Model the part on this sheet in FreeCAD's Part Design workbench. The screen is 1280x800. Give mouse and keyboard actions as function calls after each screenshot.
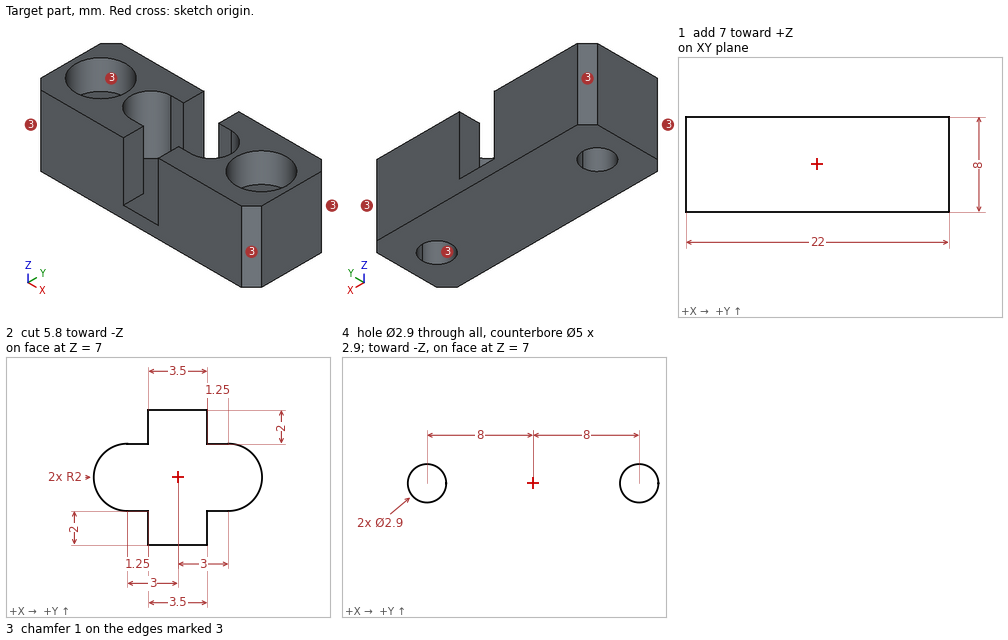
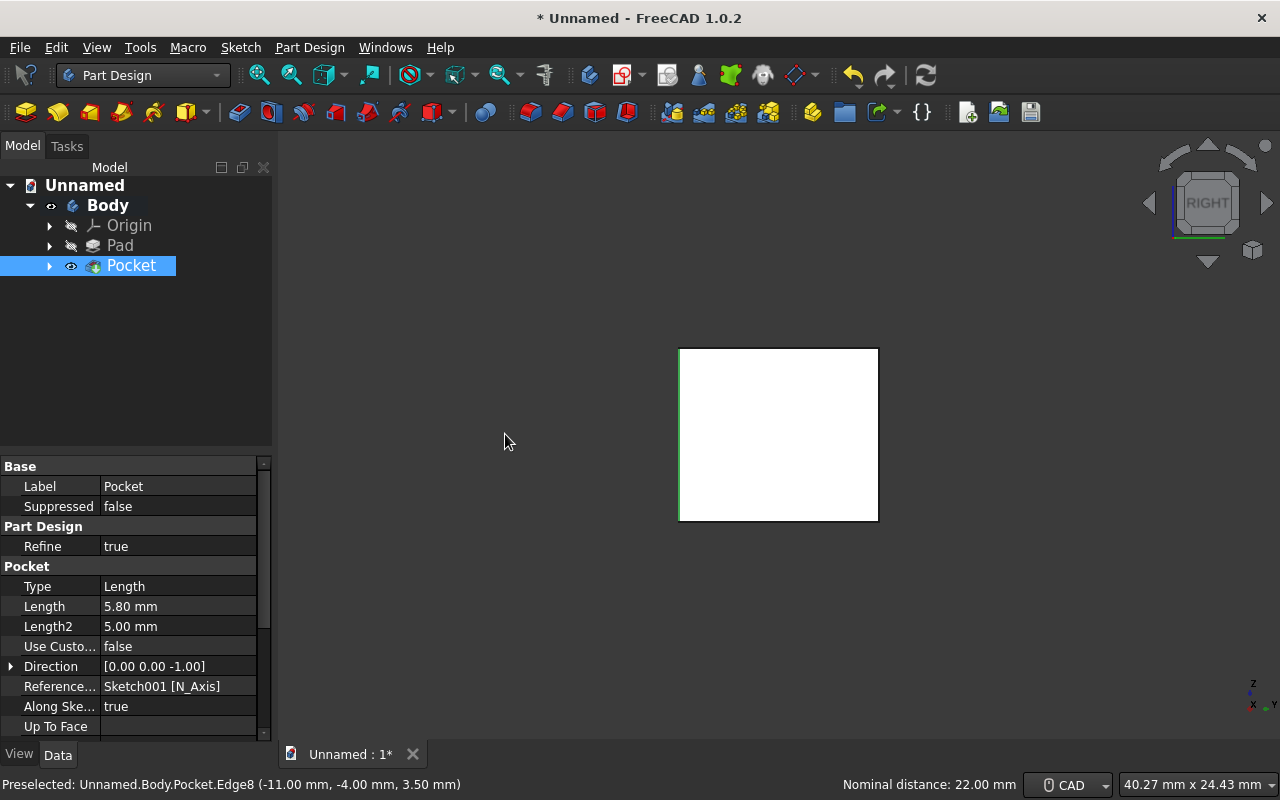
click(260, 76)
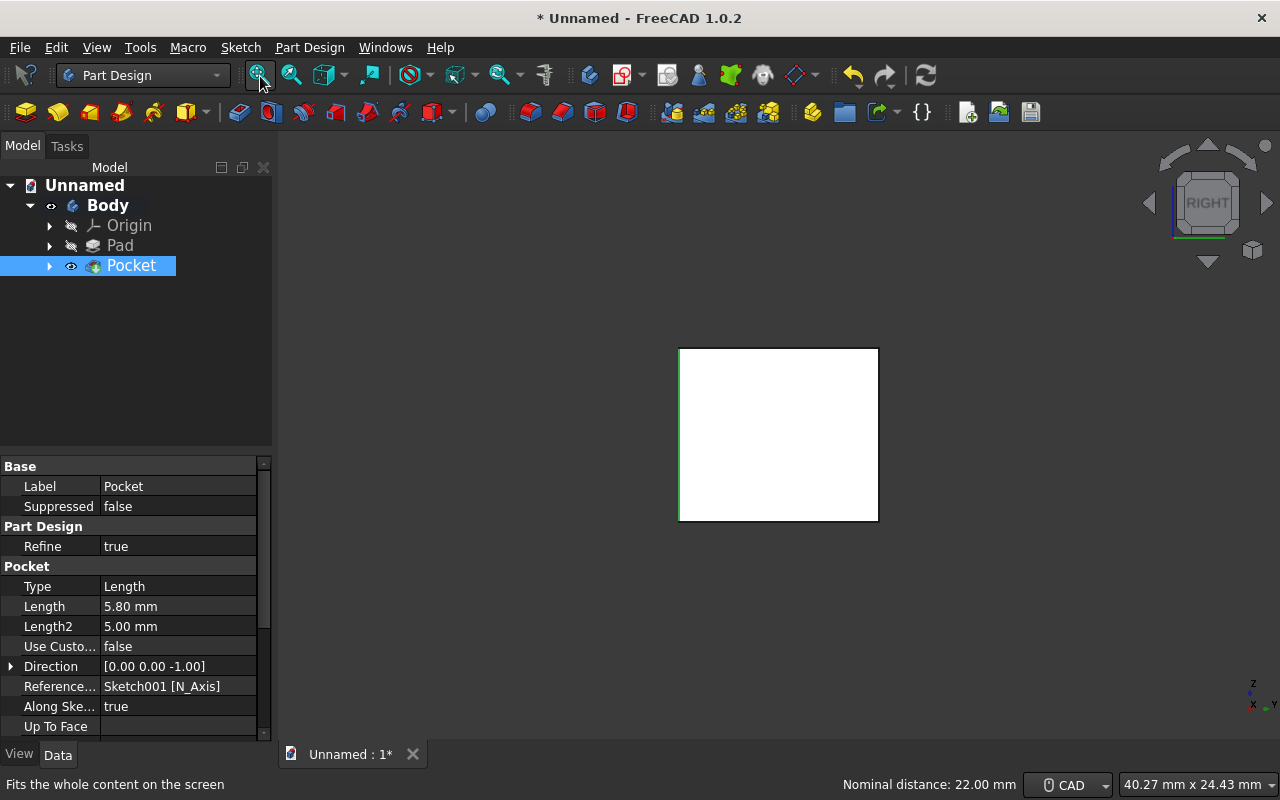
click(879, 434, ctrl)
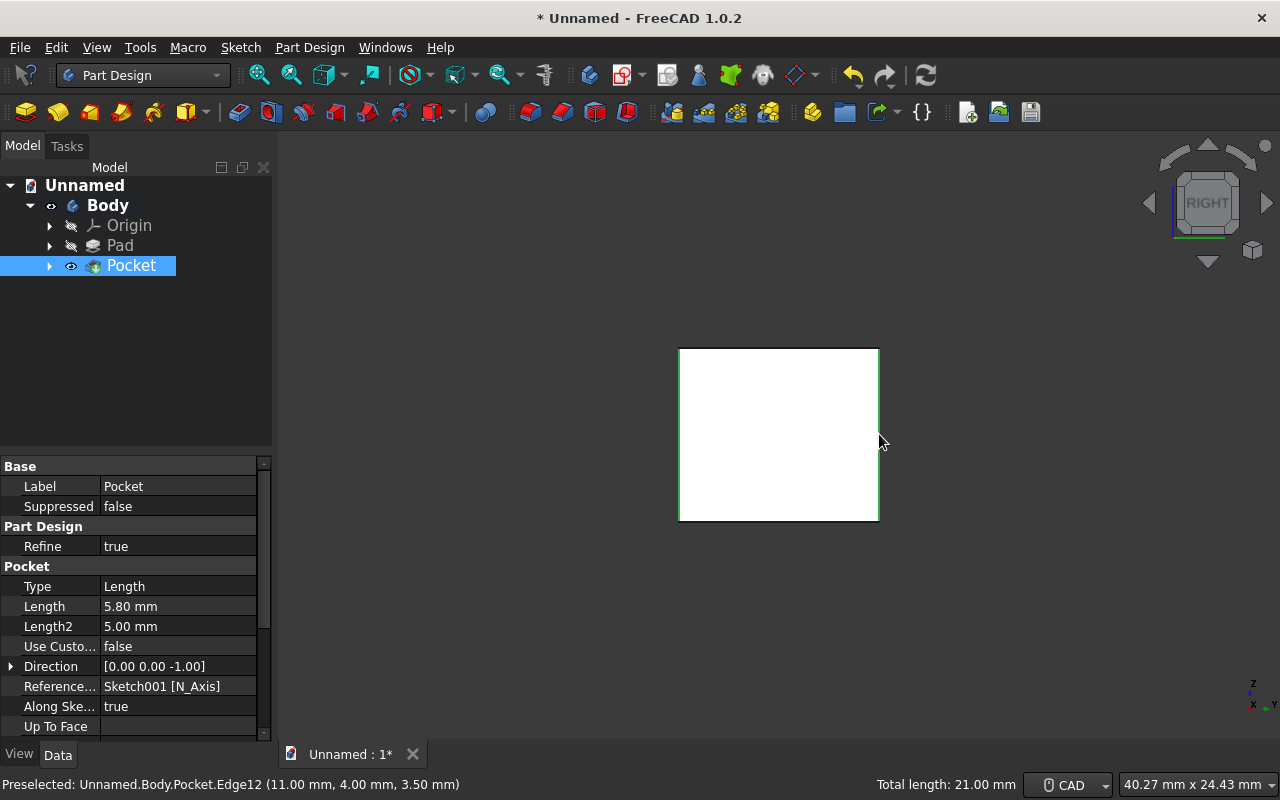
key(5)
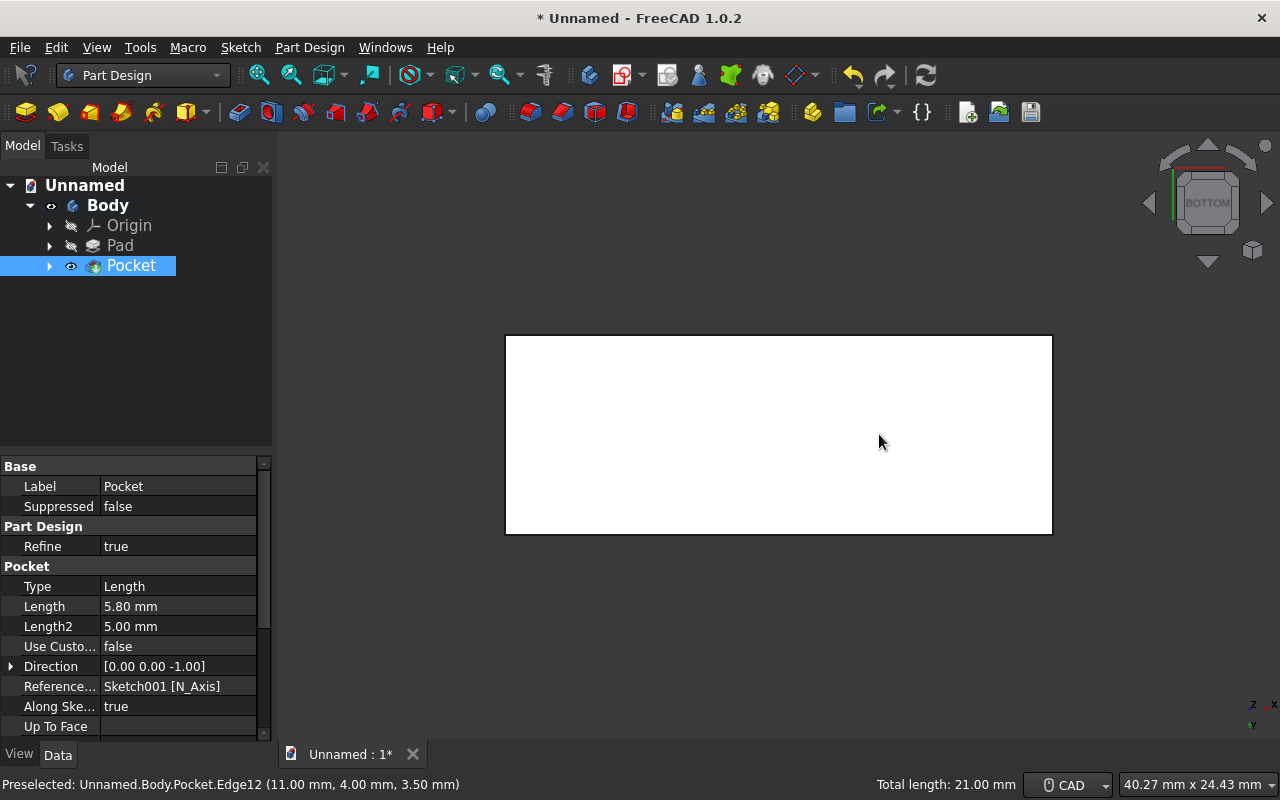
key(4)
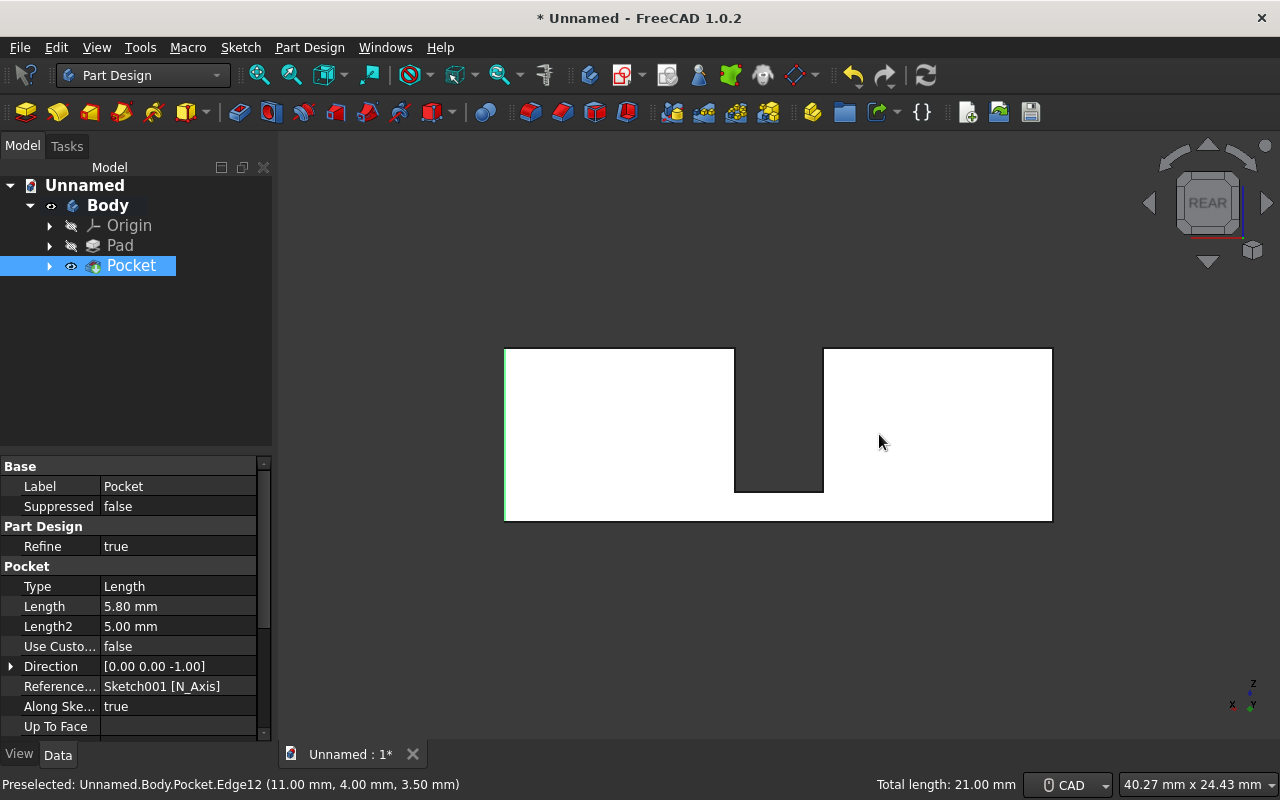
click(1053, 434, ctrl)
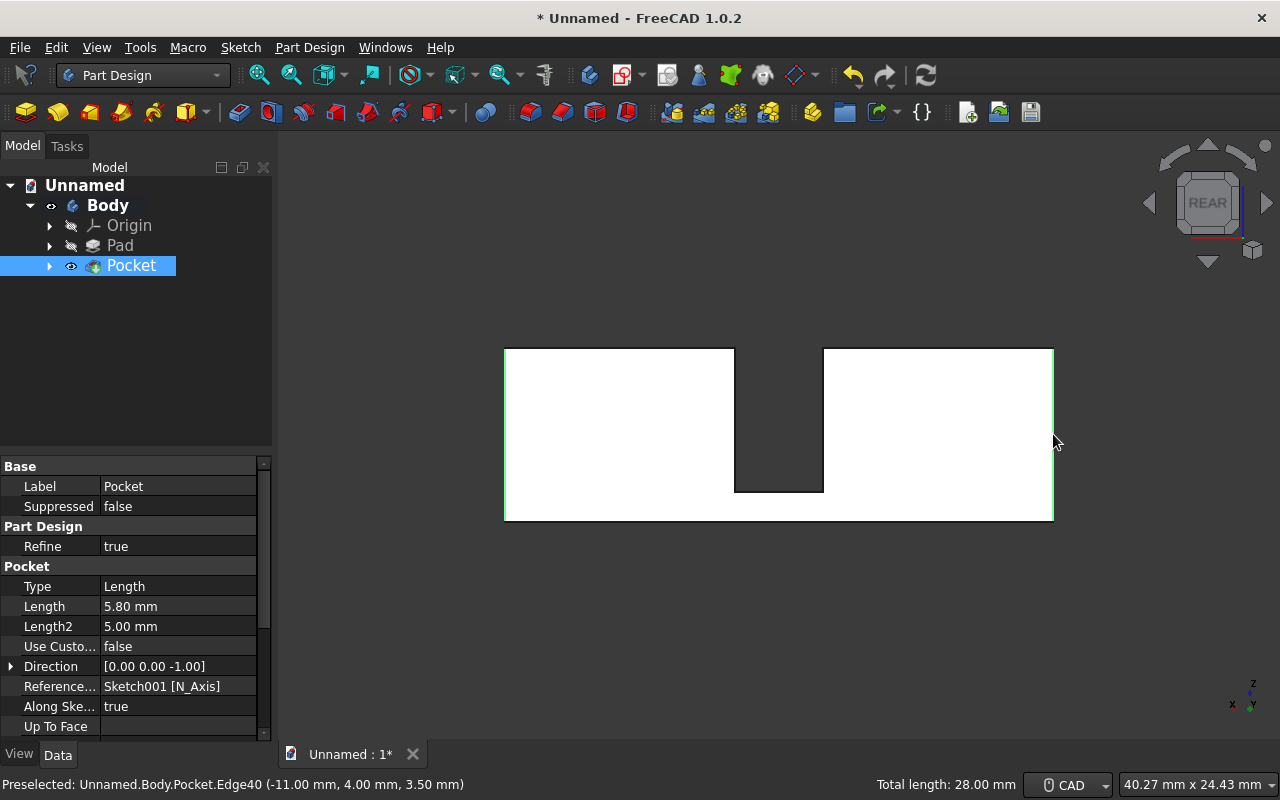
click(564, 112)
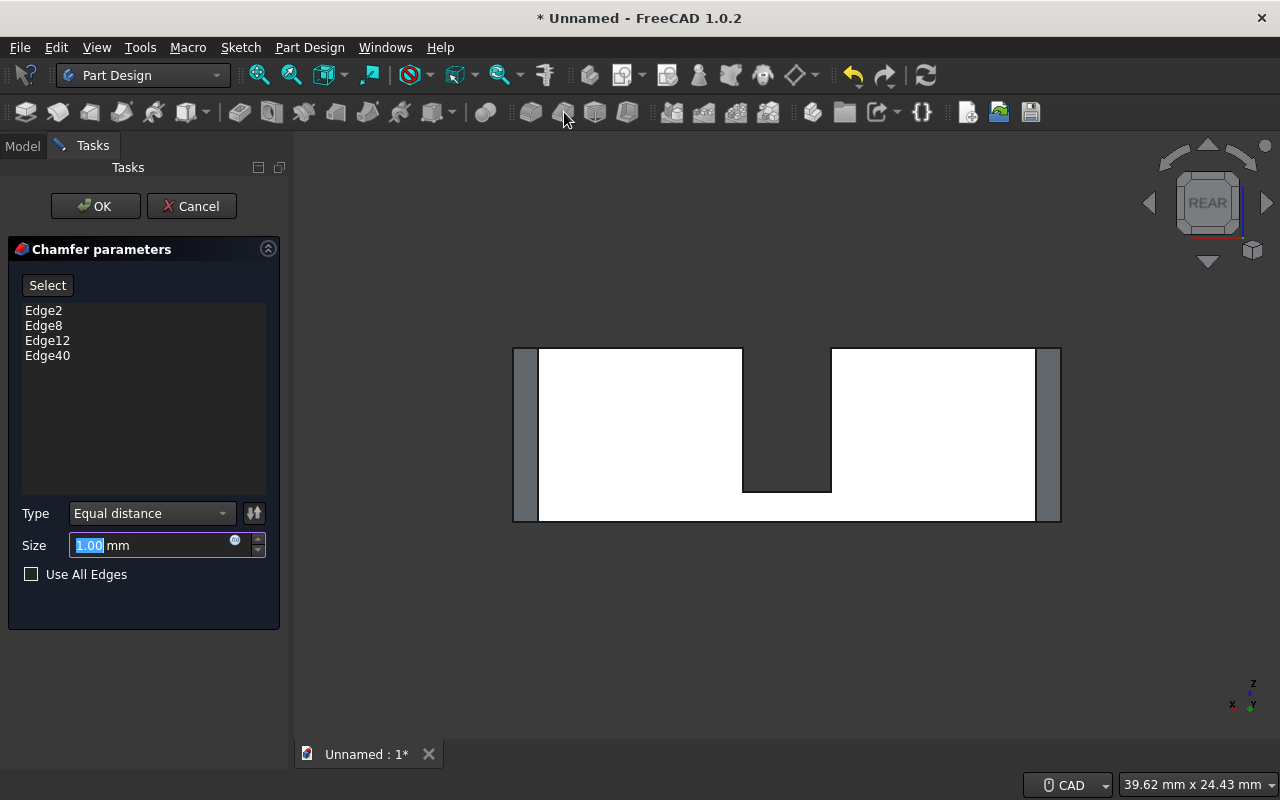
text(1)
key(Tab)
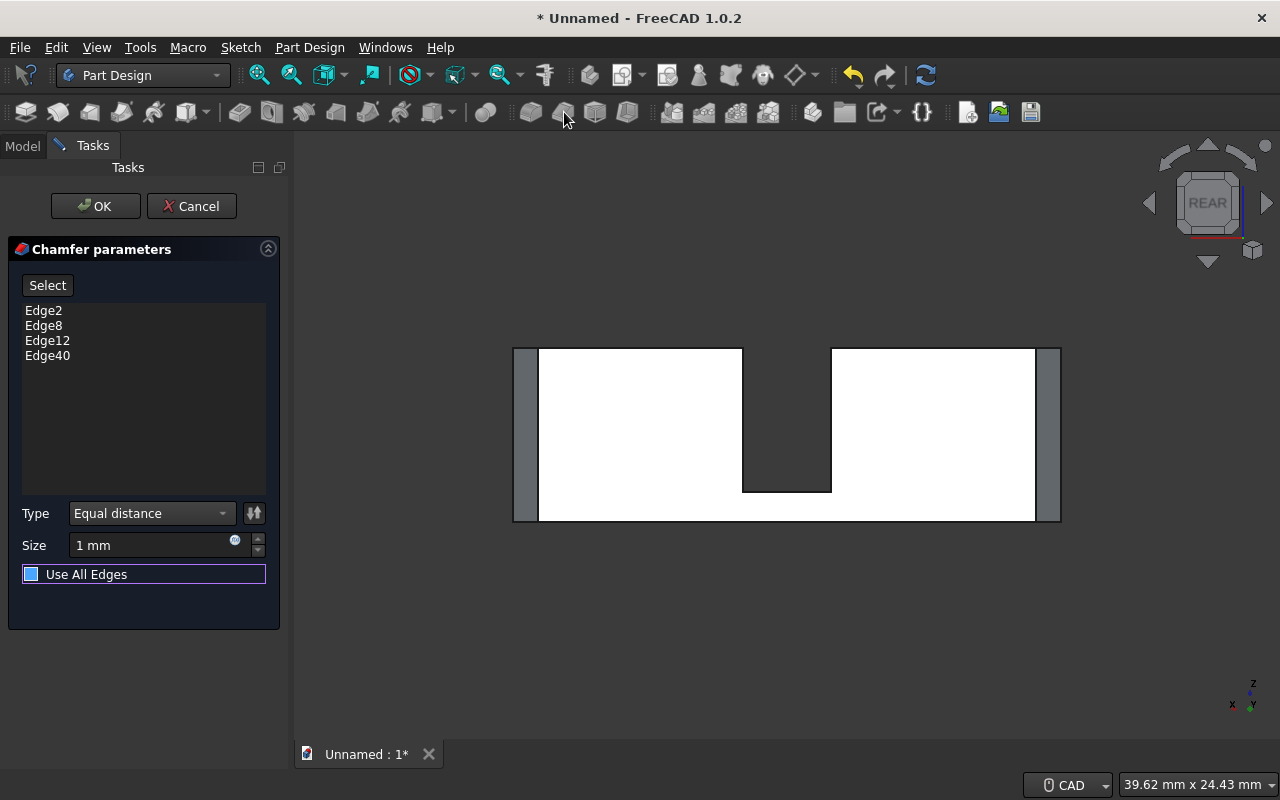
click(96, 206)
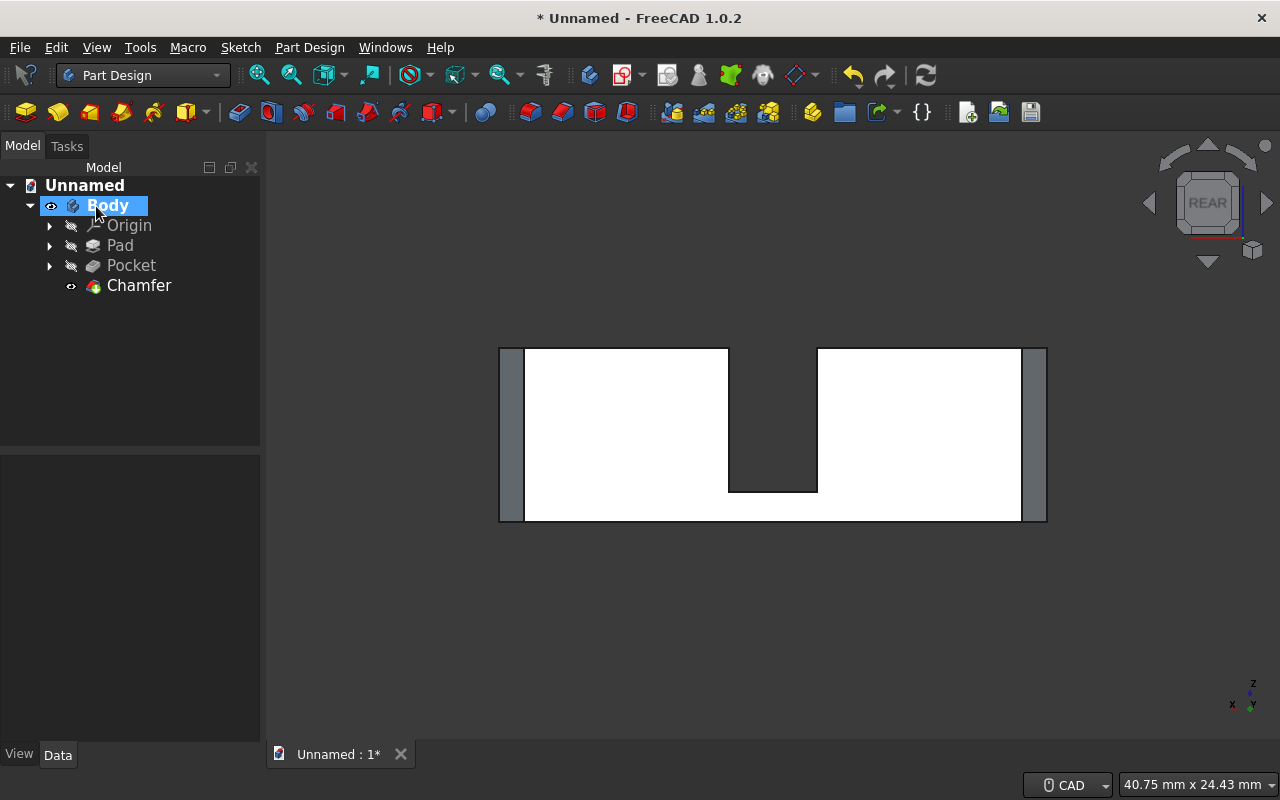
key(0)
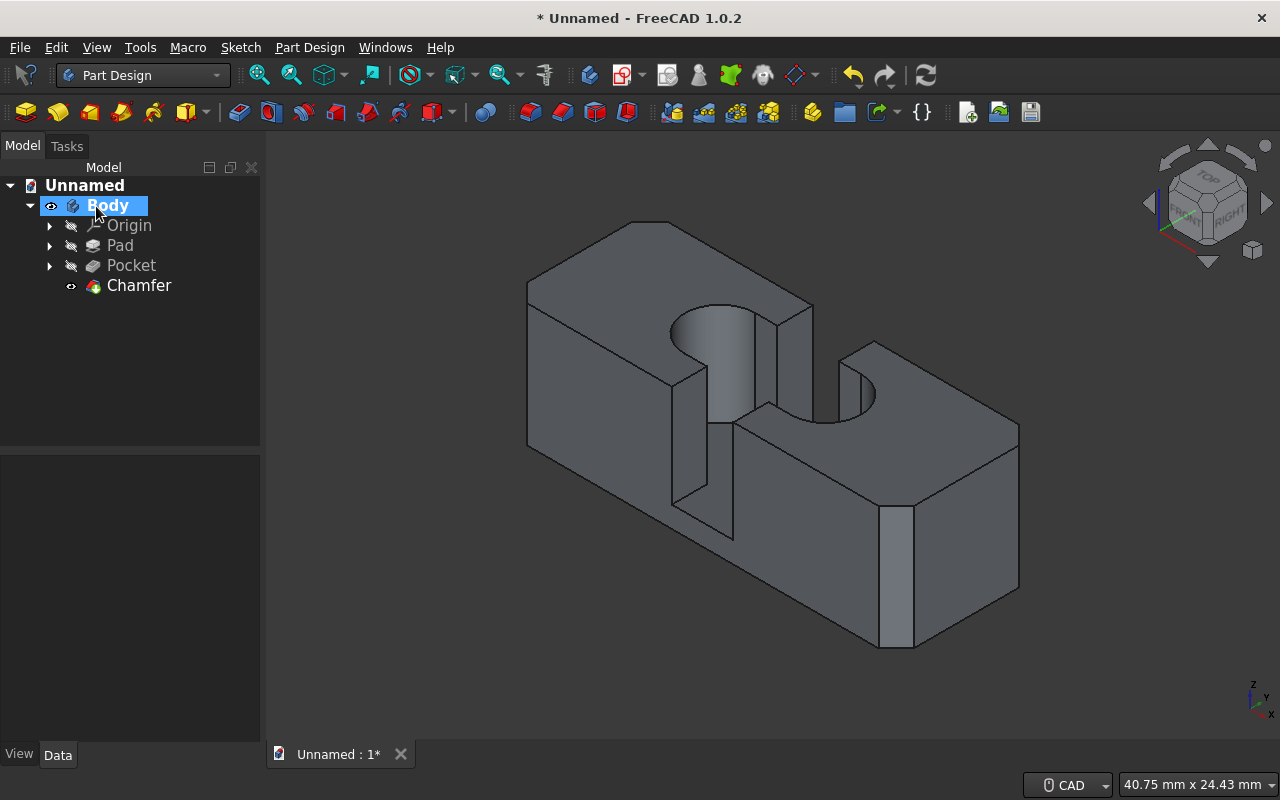
click(929, 429)